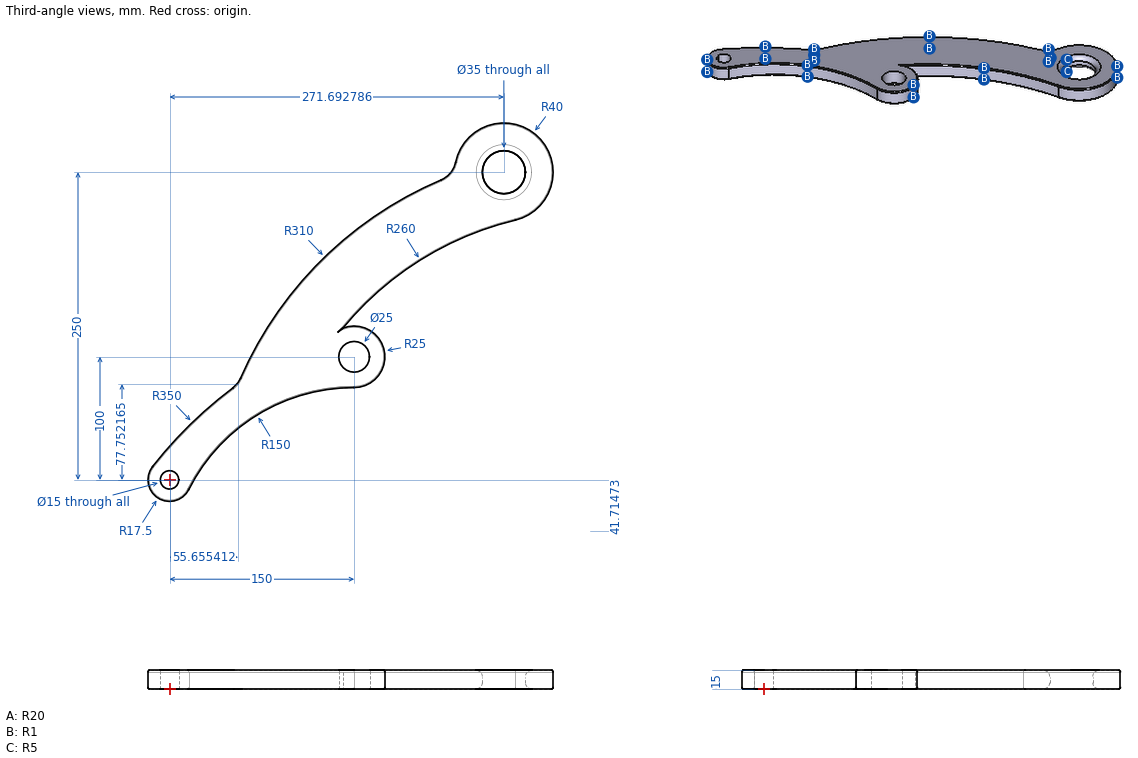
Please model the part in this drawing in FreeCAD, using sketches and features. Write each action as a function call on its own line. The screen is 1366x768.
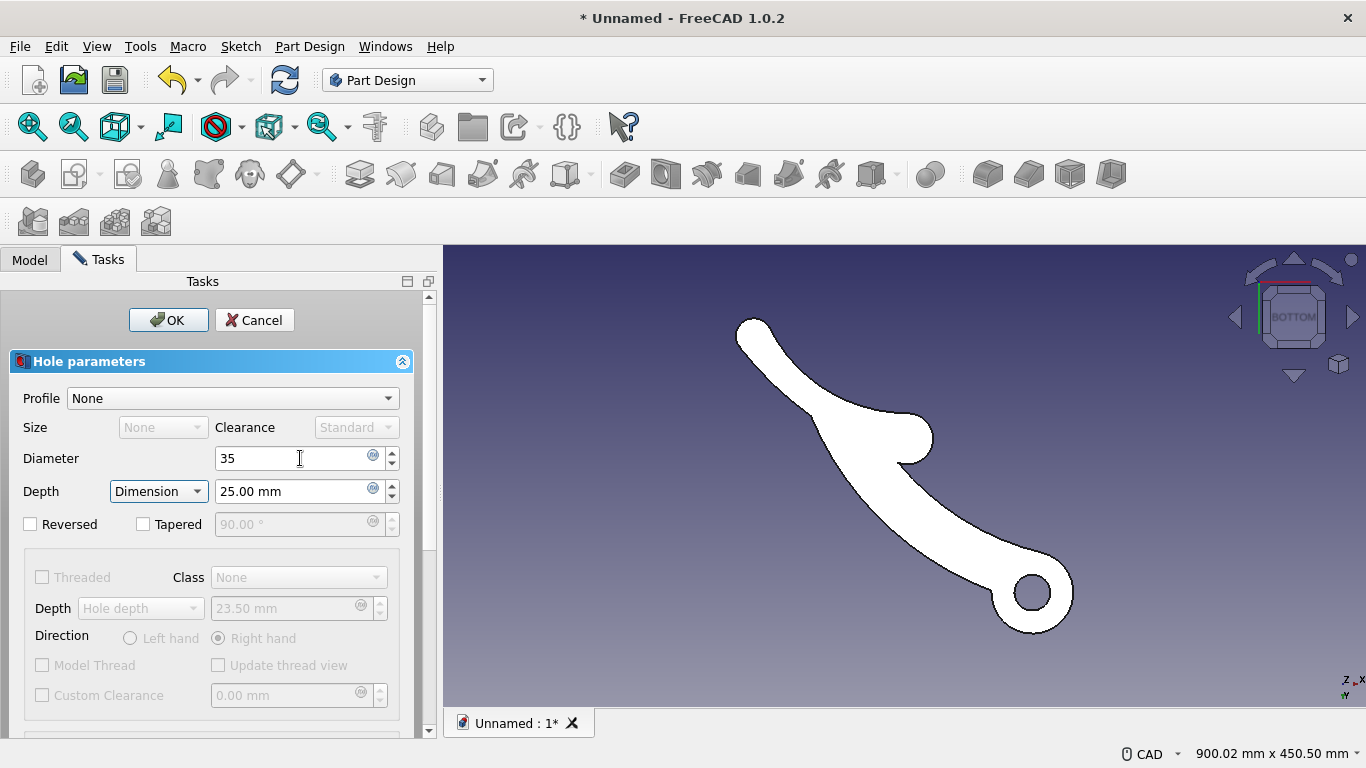
click(160, 492)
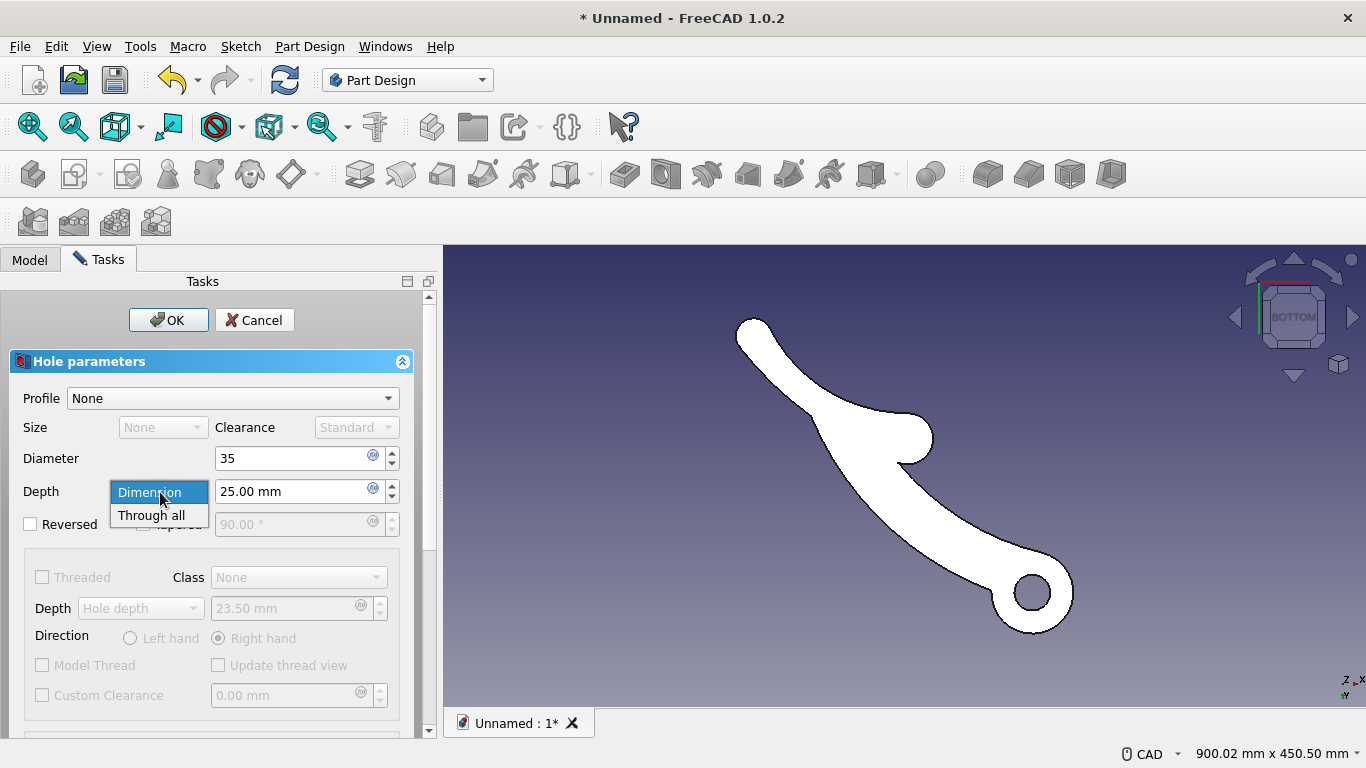
click(158, 516)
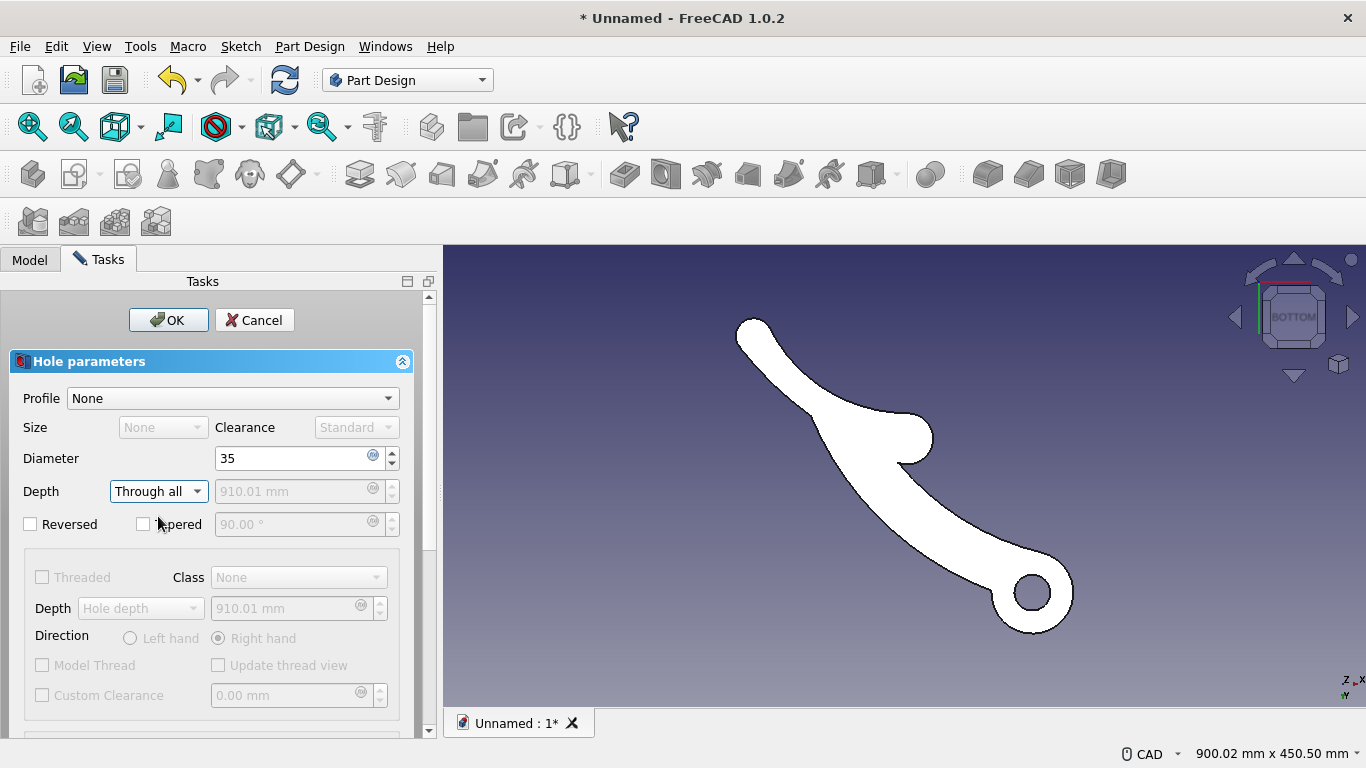
click(169, 320)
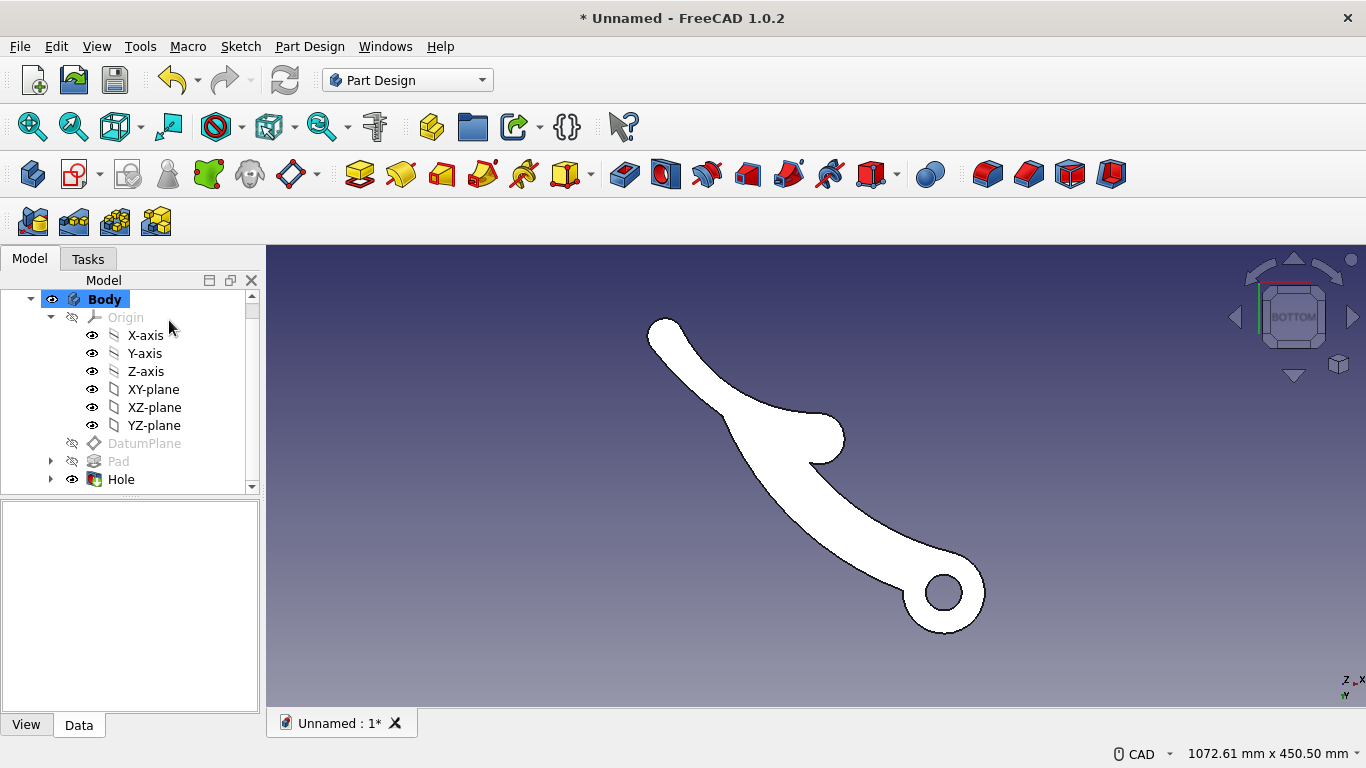
click(768, 430)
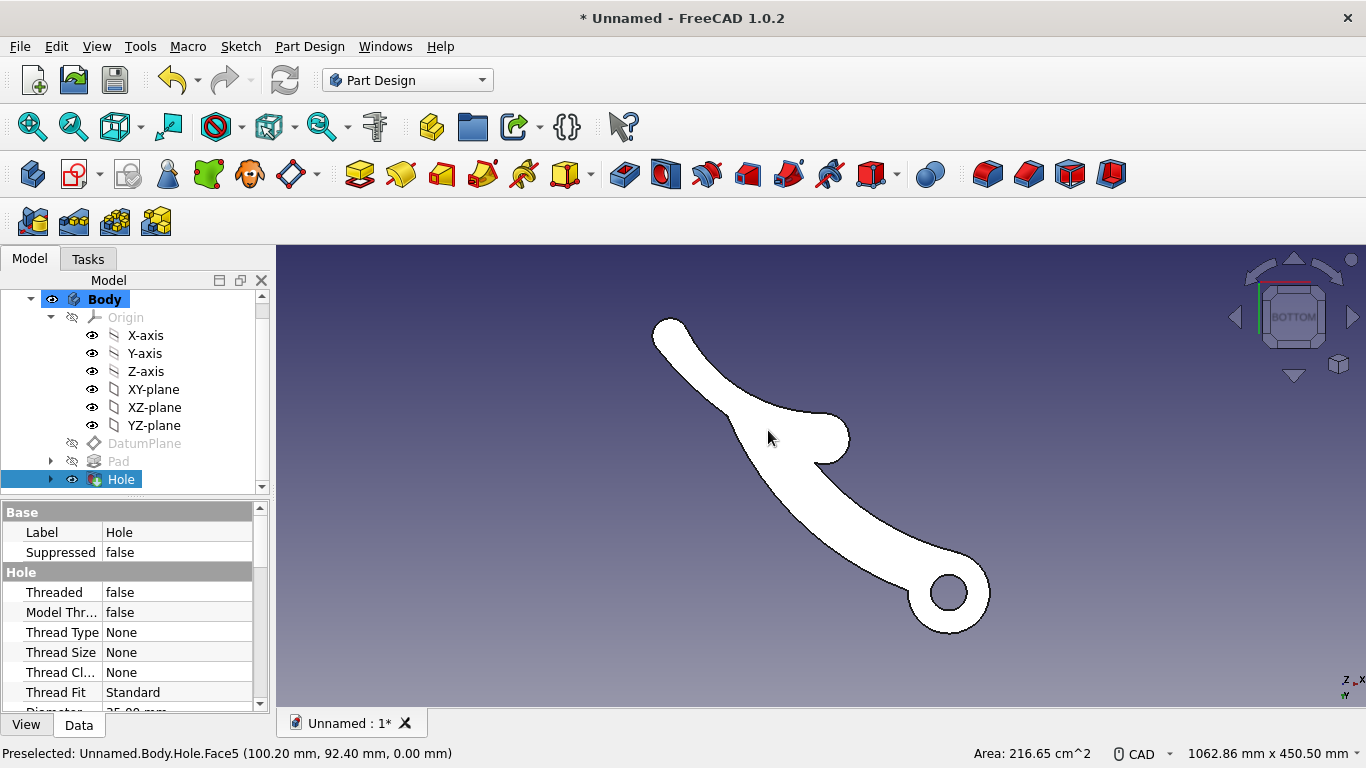
click(74, 174)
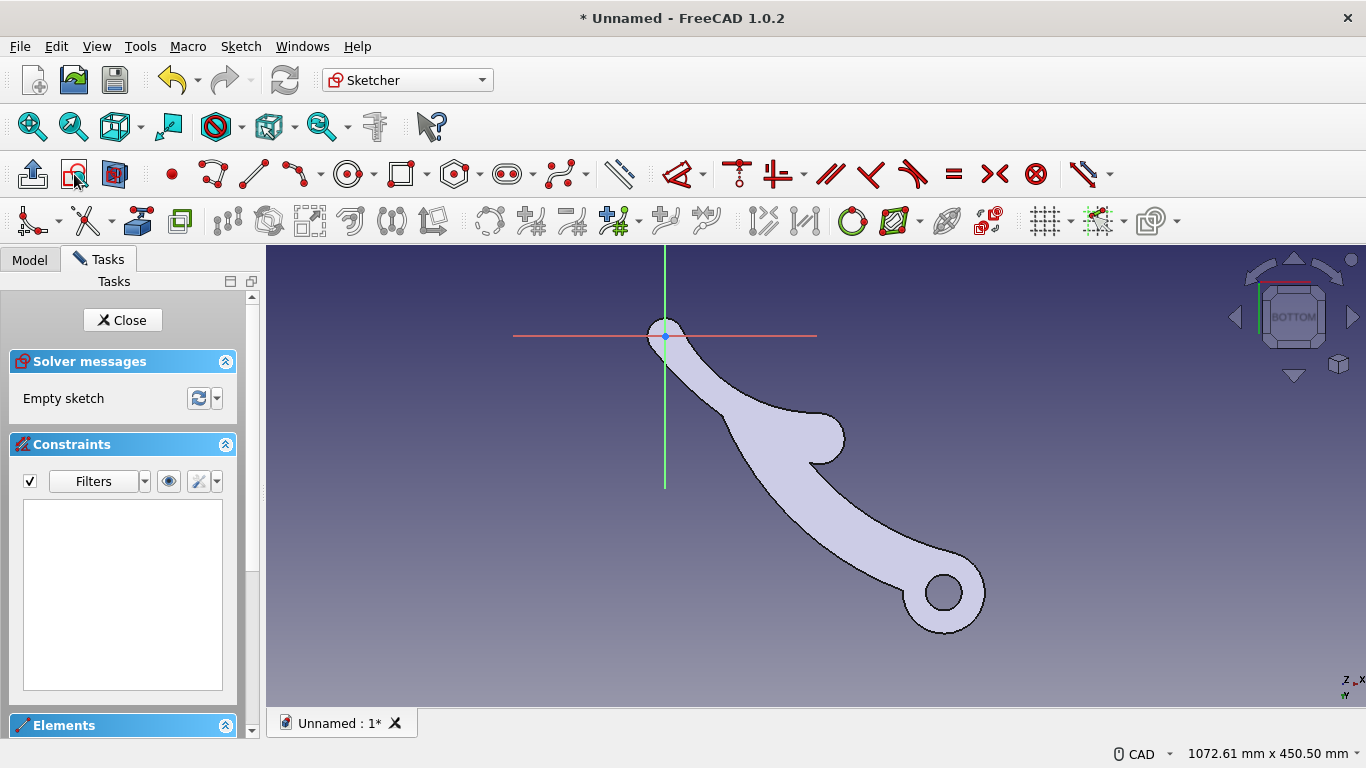
scroll(826, 435, up, 12)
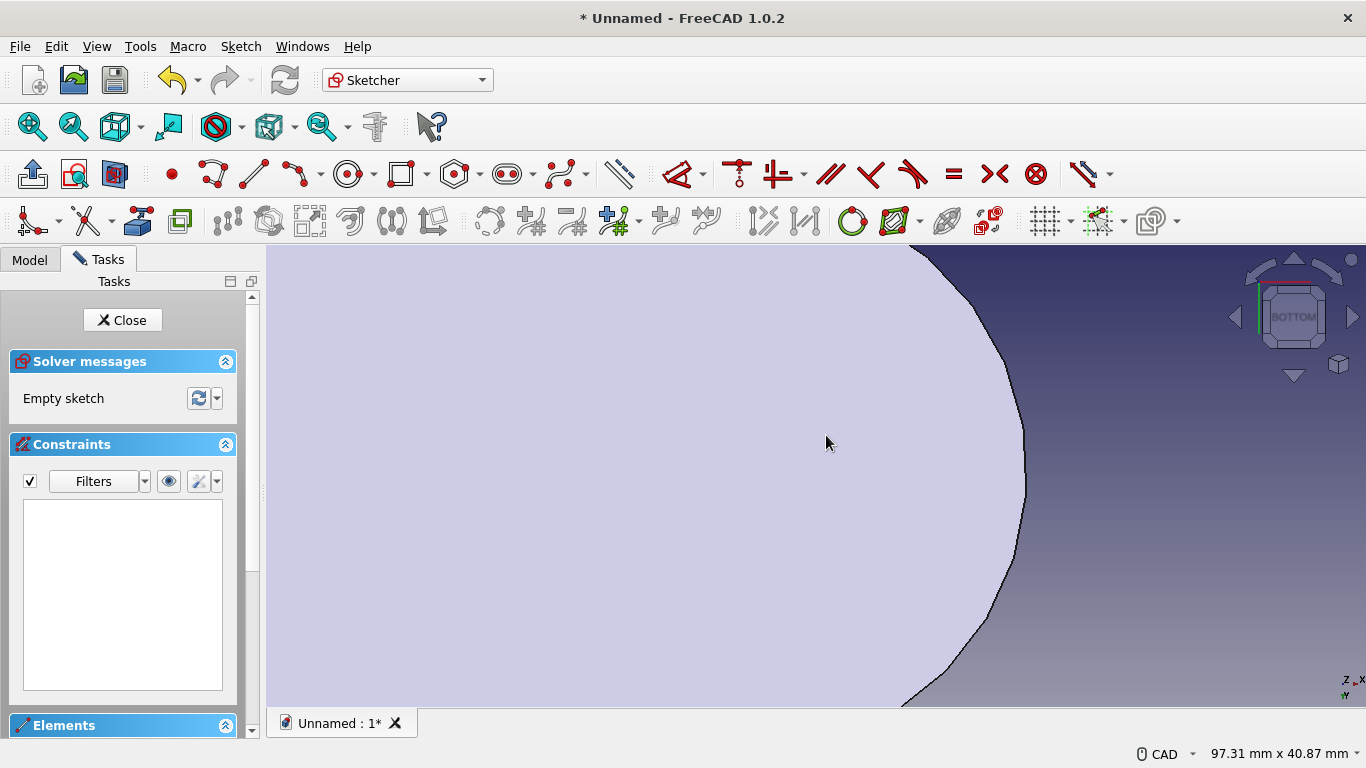
click(348, 174)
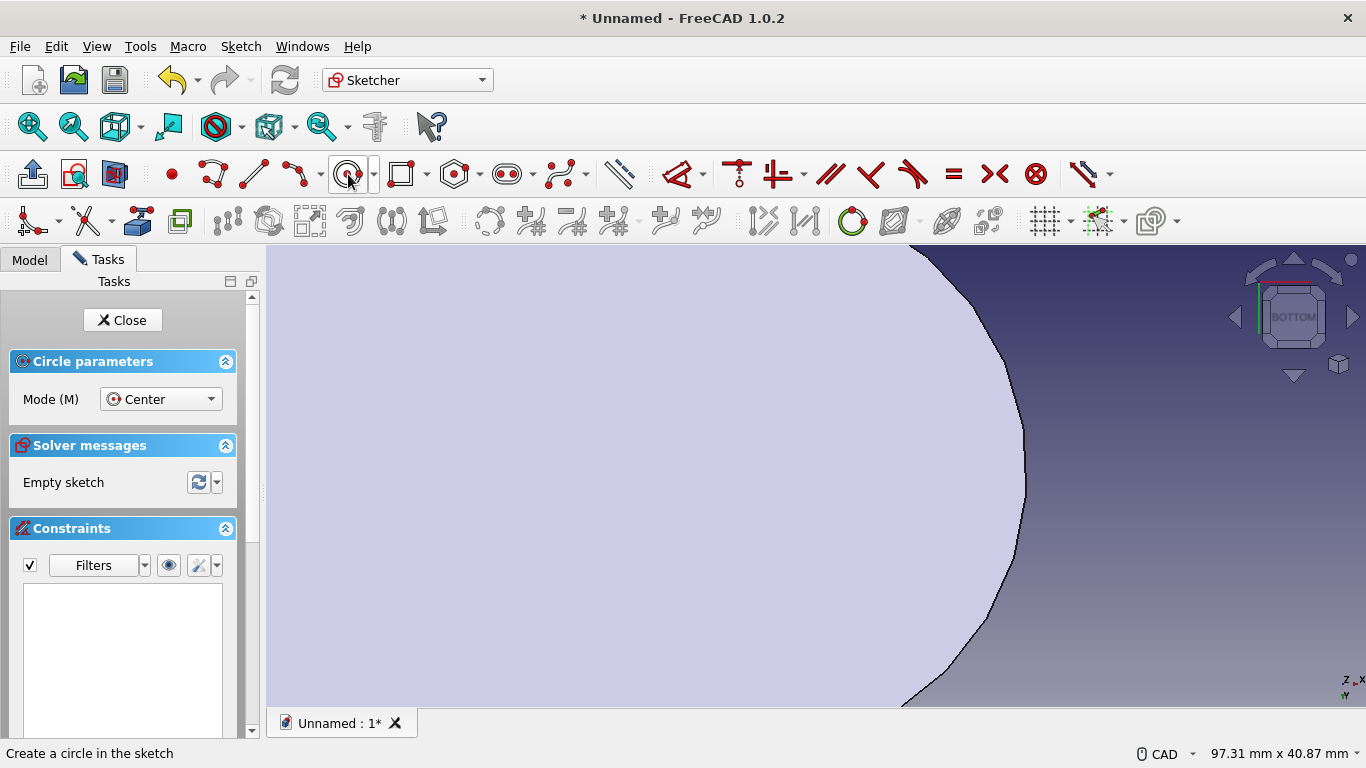
click(745, 473)
move(844, 373)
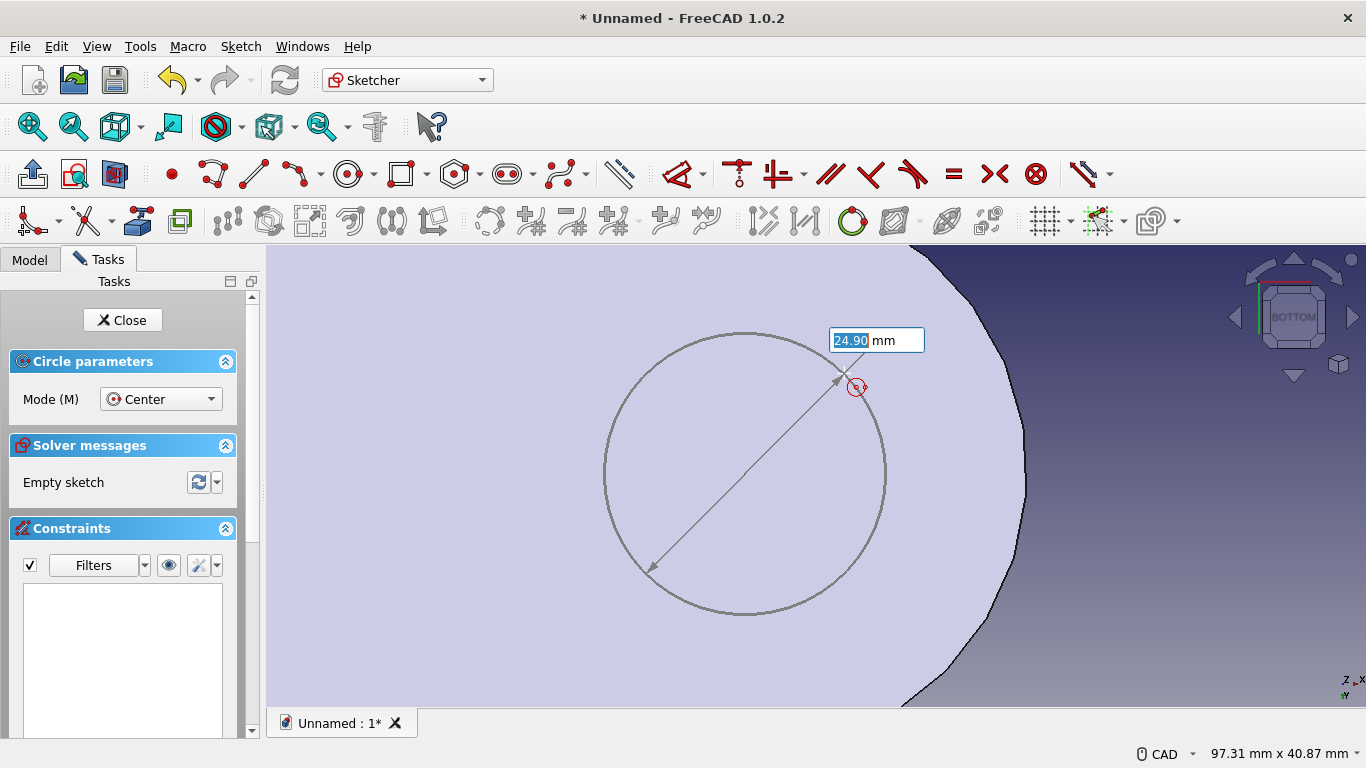
text(25)
key(Return)
key(Escape)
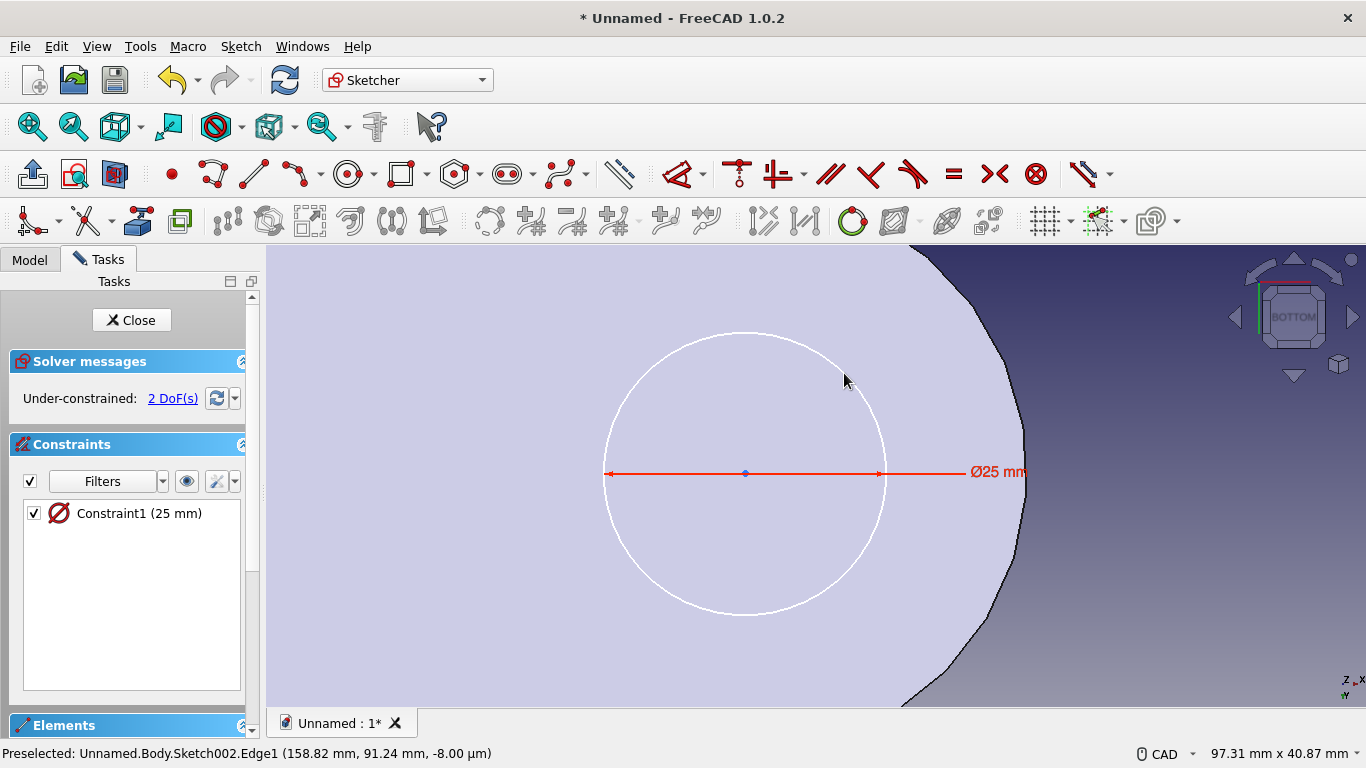
key(d)